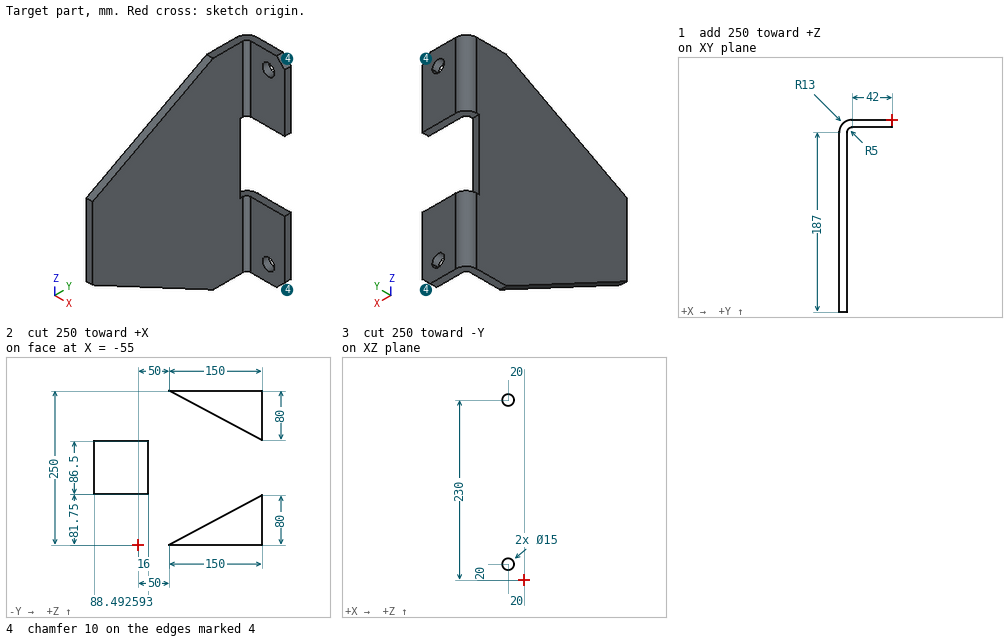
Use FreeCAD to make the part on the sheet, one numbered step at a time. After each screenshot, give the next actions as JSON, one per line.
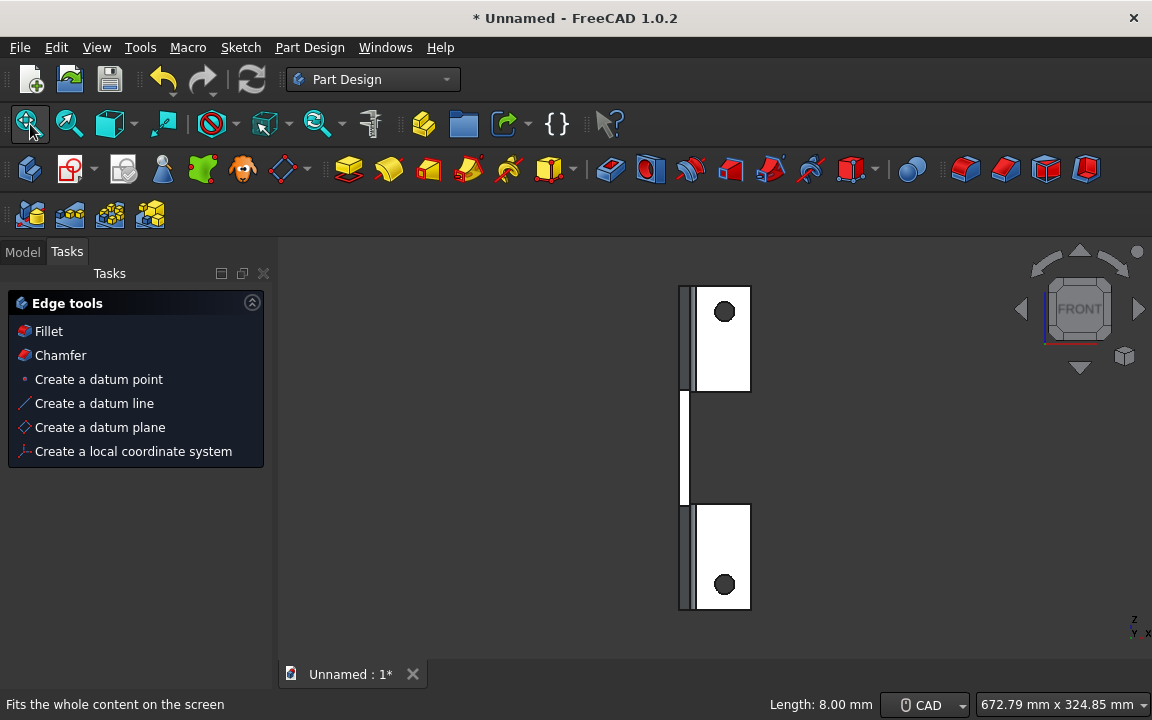
{"action": "key", "text": "3"}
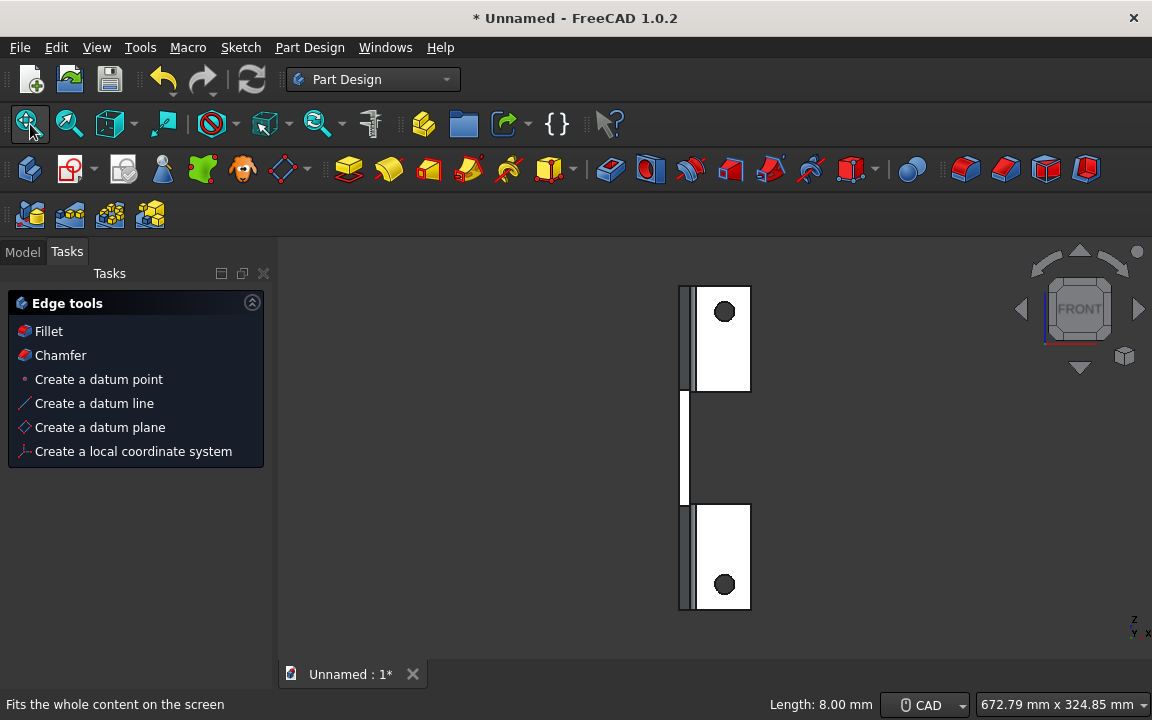
{"action": "scroll", "coordinate": [840, 609], "scroll_direction": "up", "scroll_amount": 7}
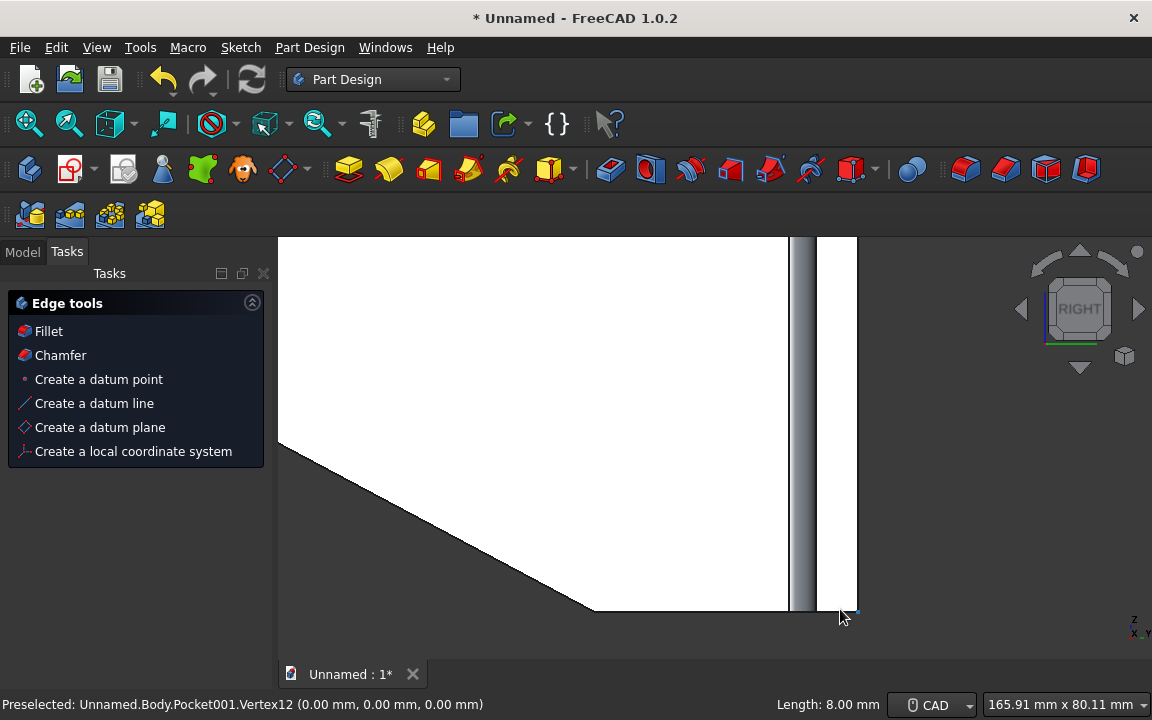
{"action": "left_click", "coordinate": [837, 611], "text": "ctrl"}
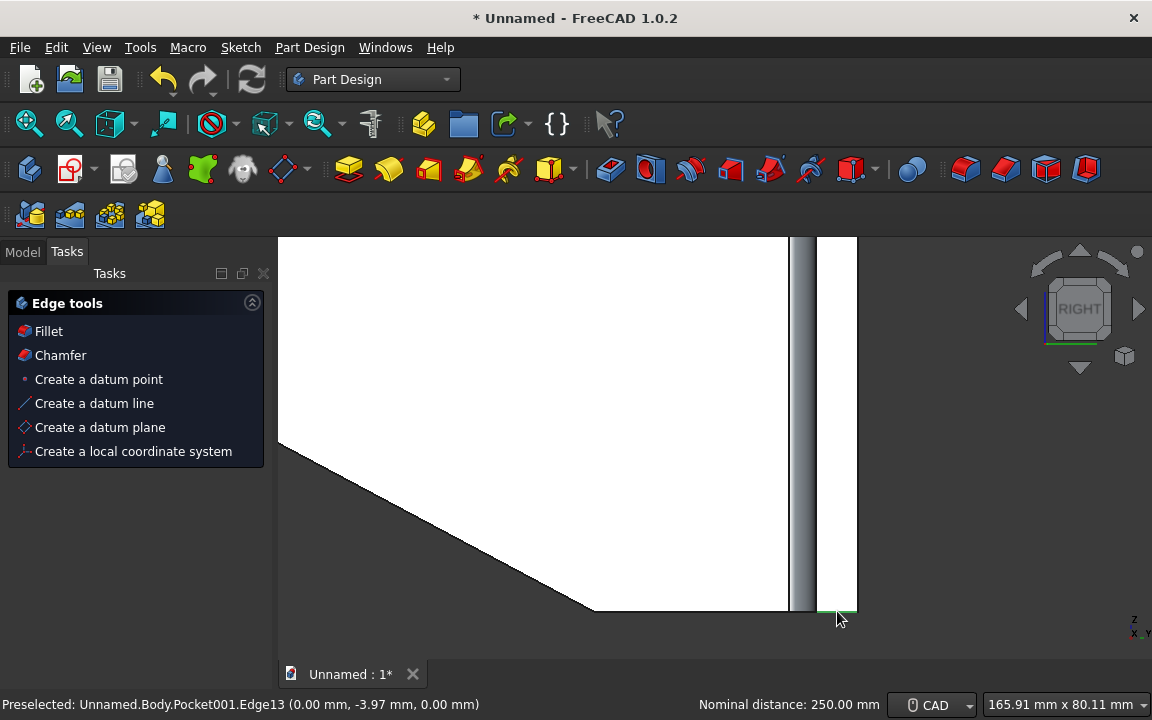
{"action": "left_click", "coordinate": [1006, 170]}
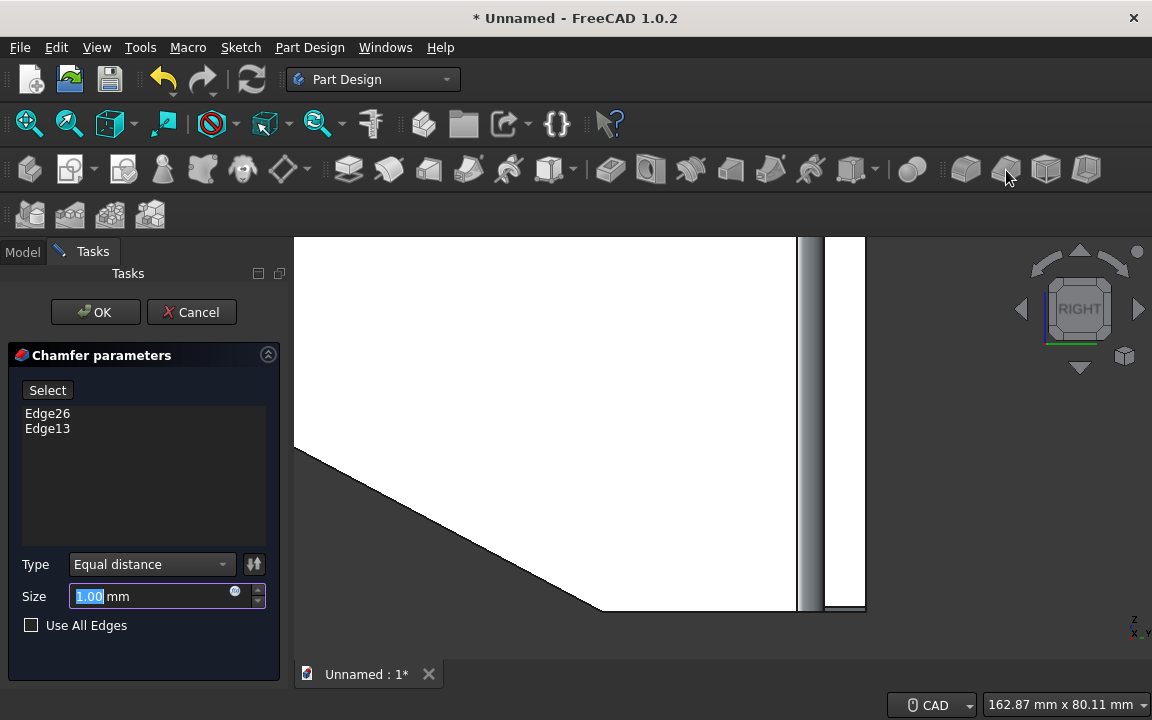
{"action": "type", "text": "10"}
{"action": "key", "text": "Tab"}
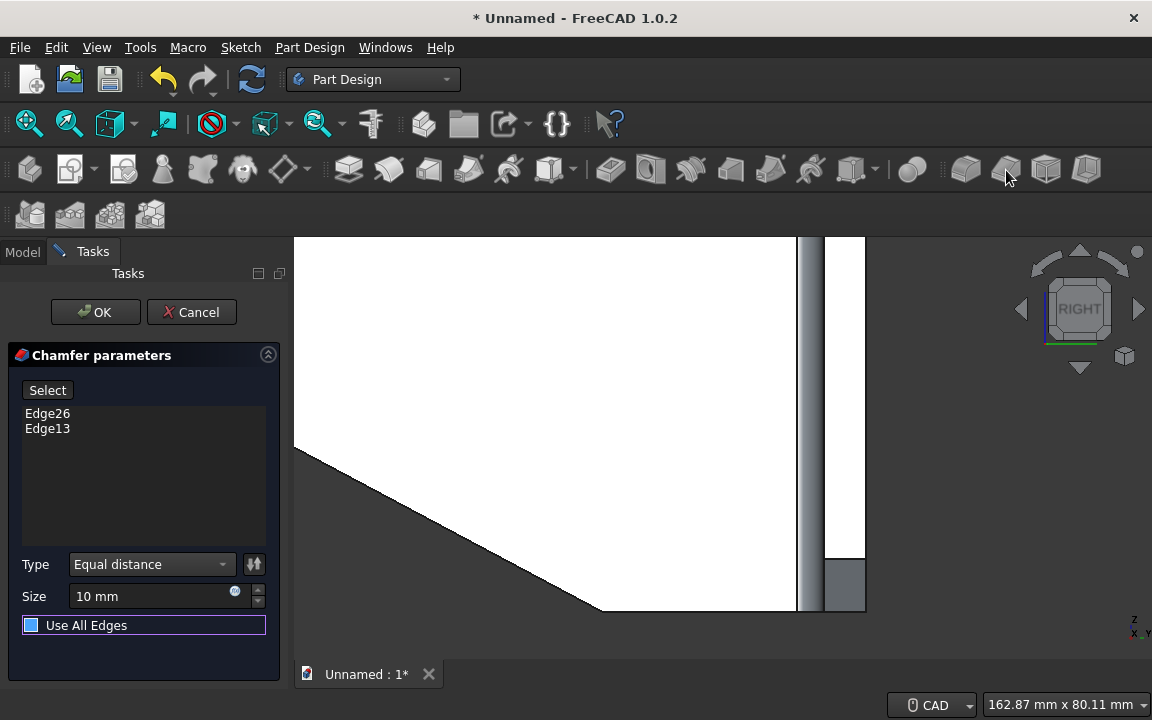
{"action": "left_click", "coordinate": [96, 312]}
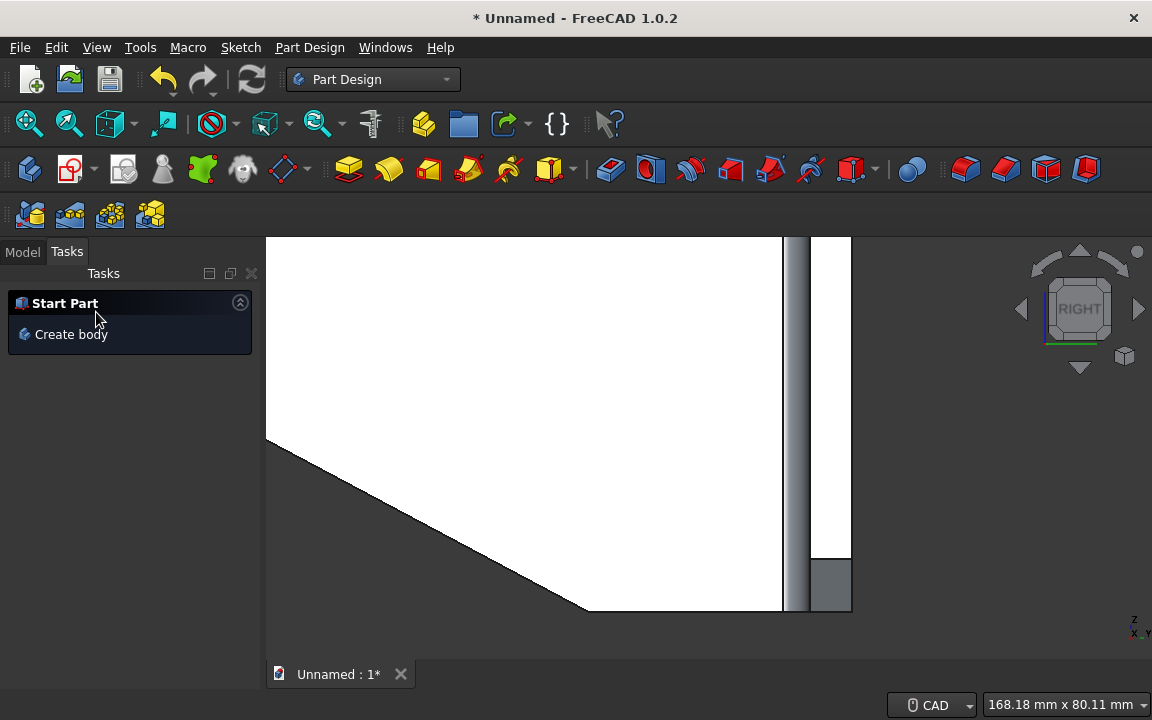
{"action": "key", "text": "0"}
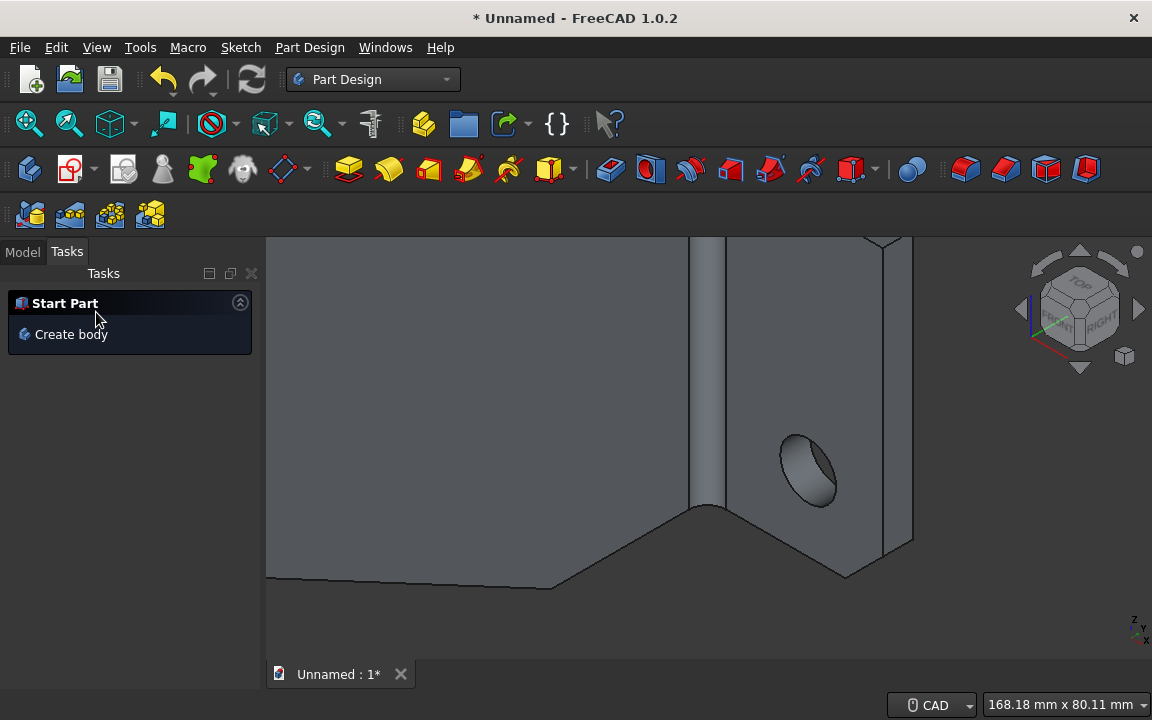
{"action": "left_click", "coordinate": [30, 124]}